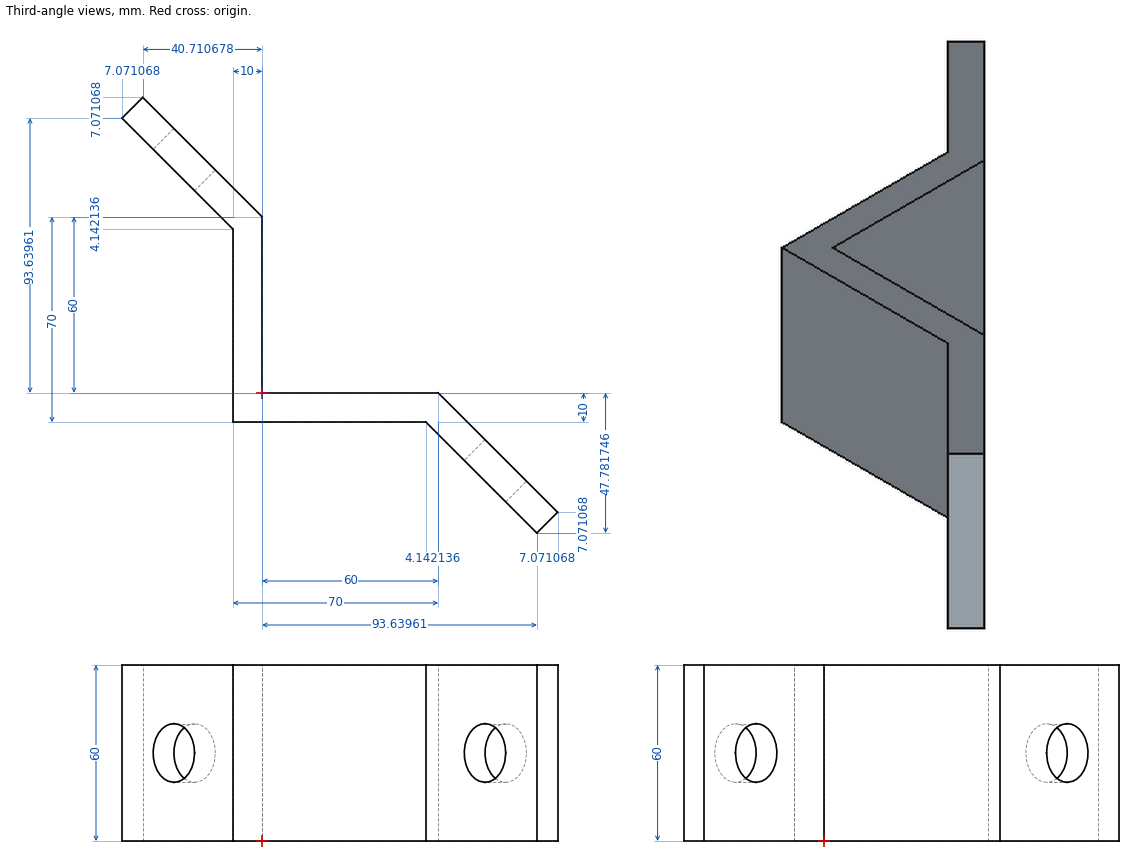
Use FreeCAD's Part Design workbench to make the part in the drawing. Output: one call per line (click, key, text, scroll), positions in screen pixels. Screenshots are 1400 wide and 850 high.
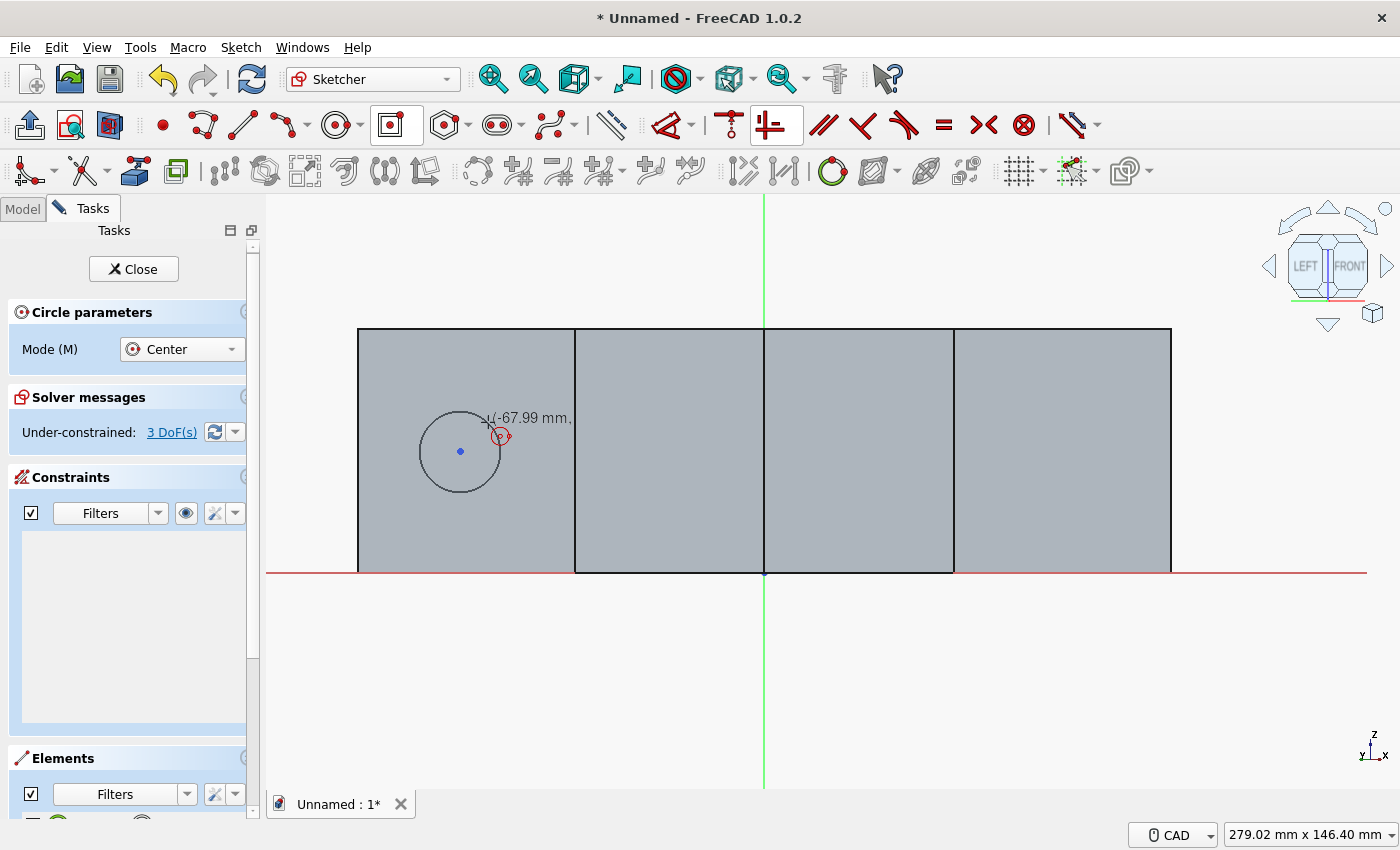
click(1069, 451)
click(1098, 422)
key(Escape)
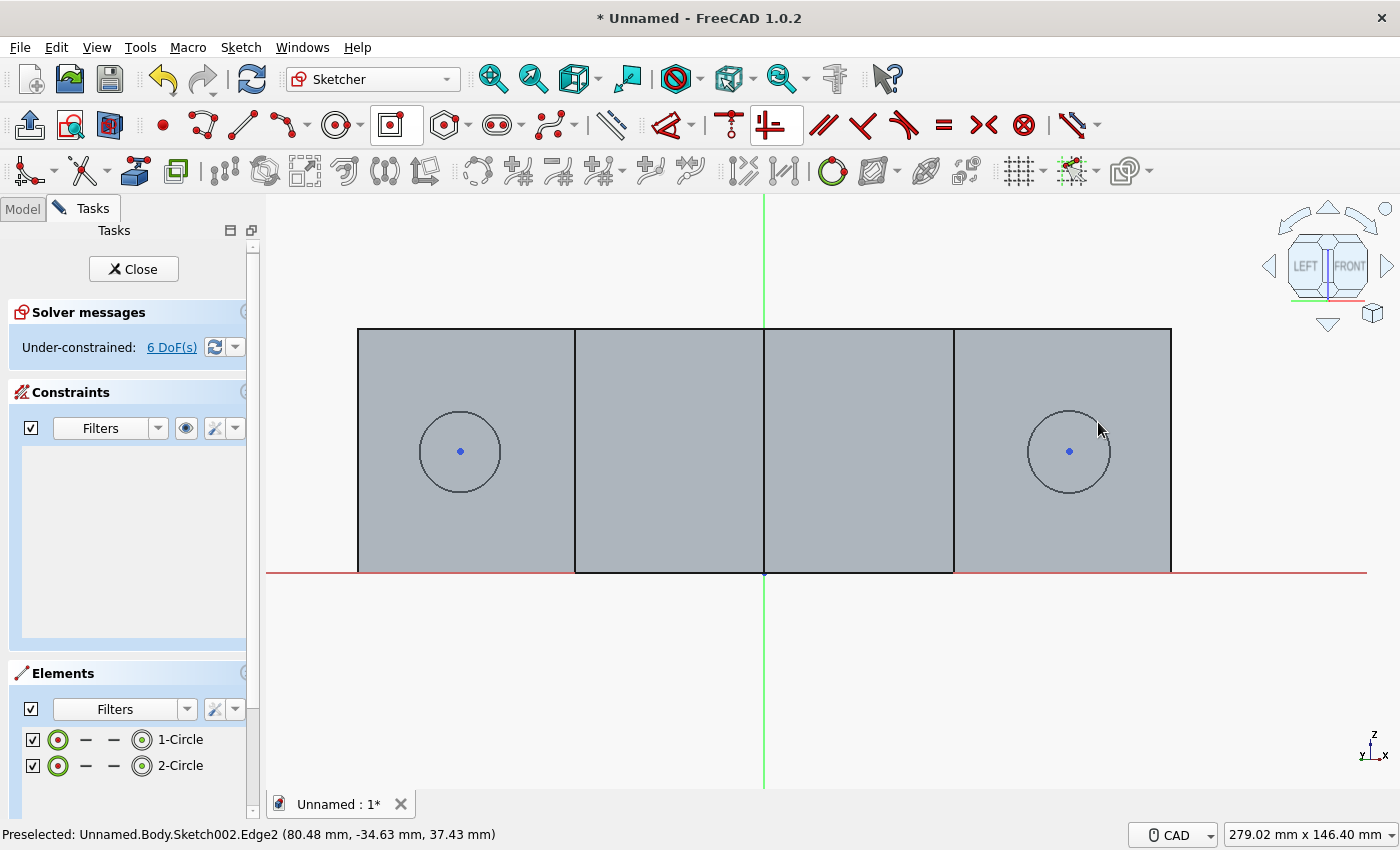
click(488, 423)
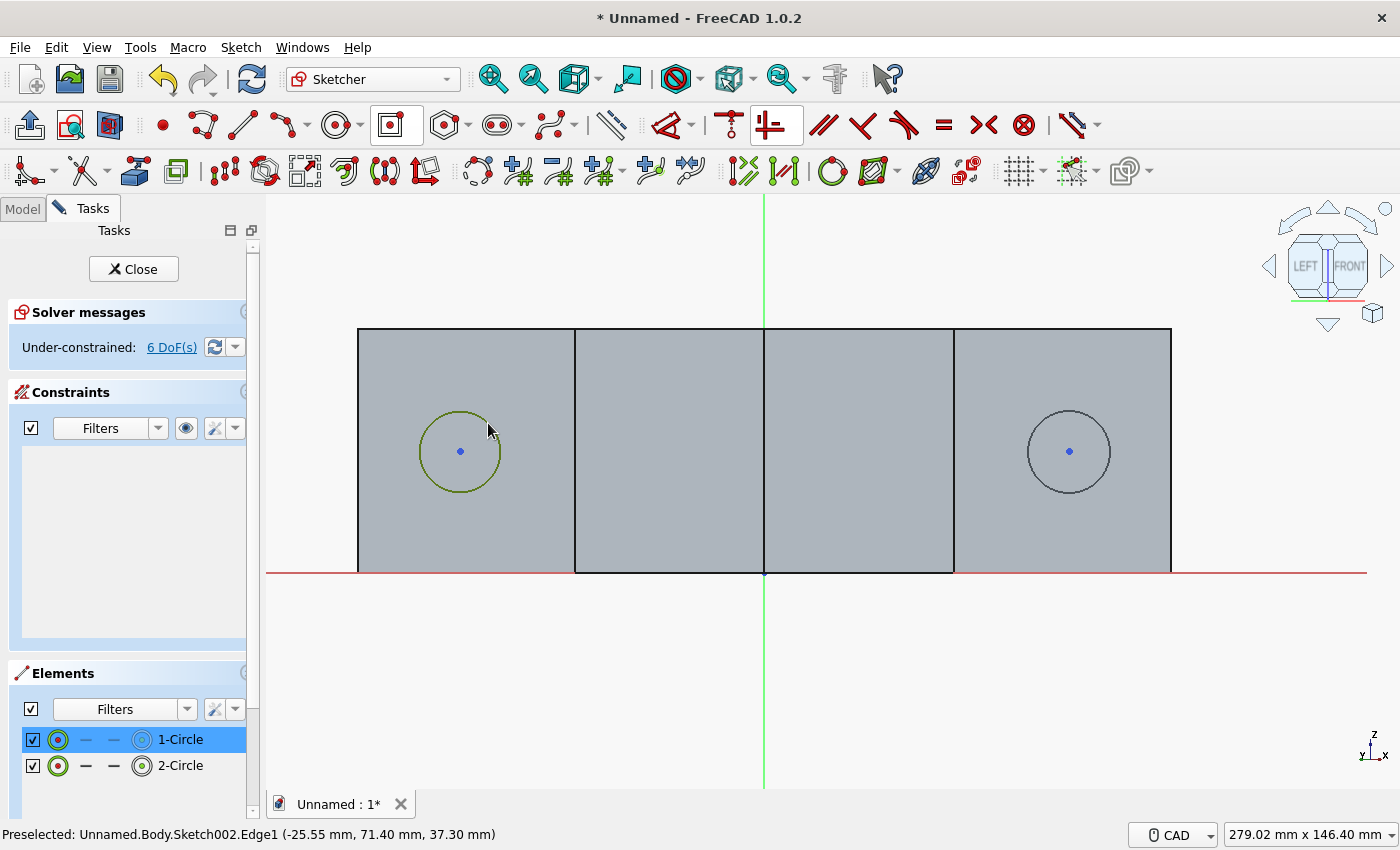
click(1098, 423)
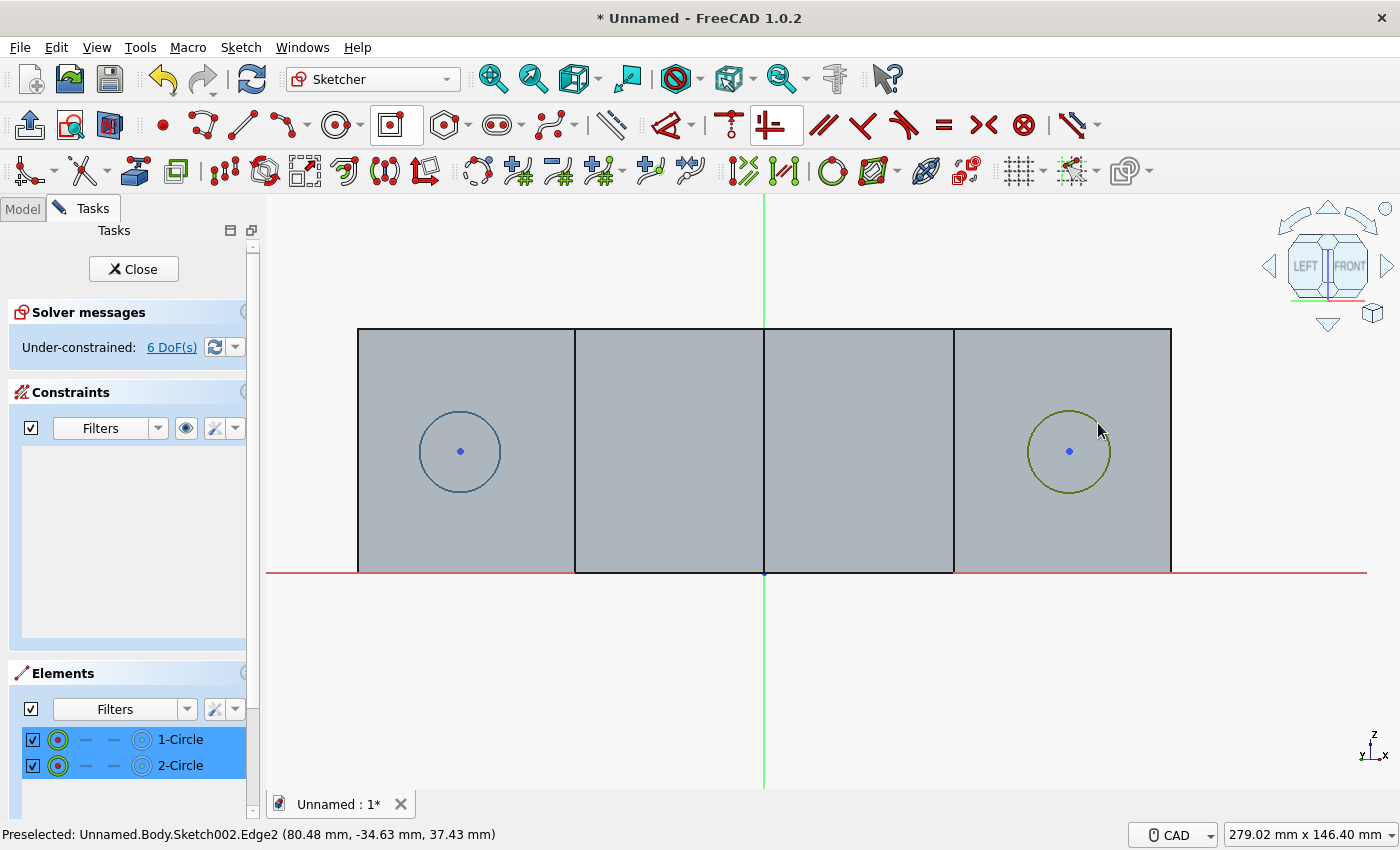
click(944, 126)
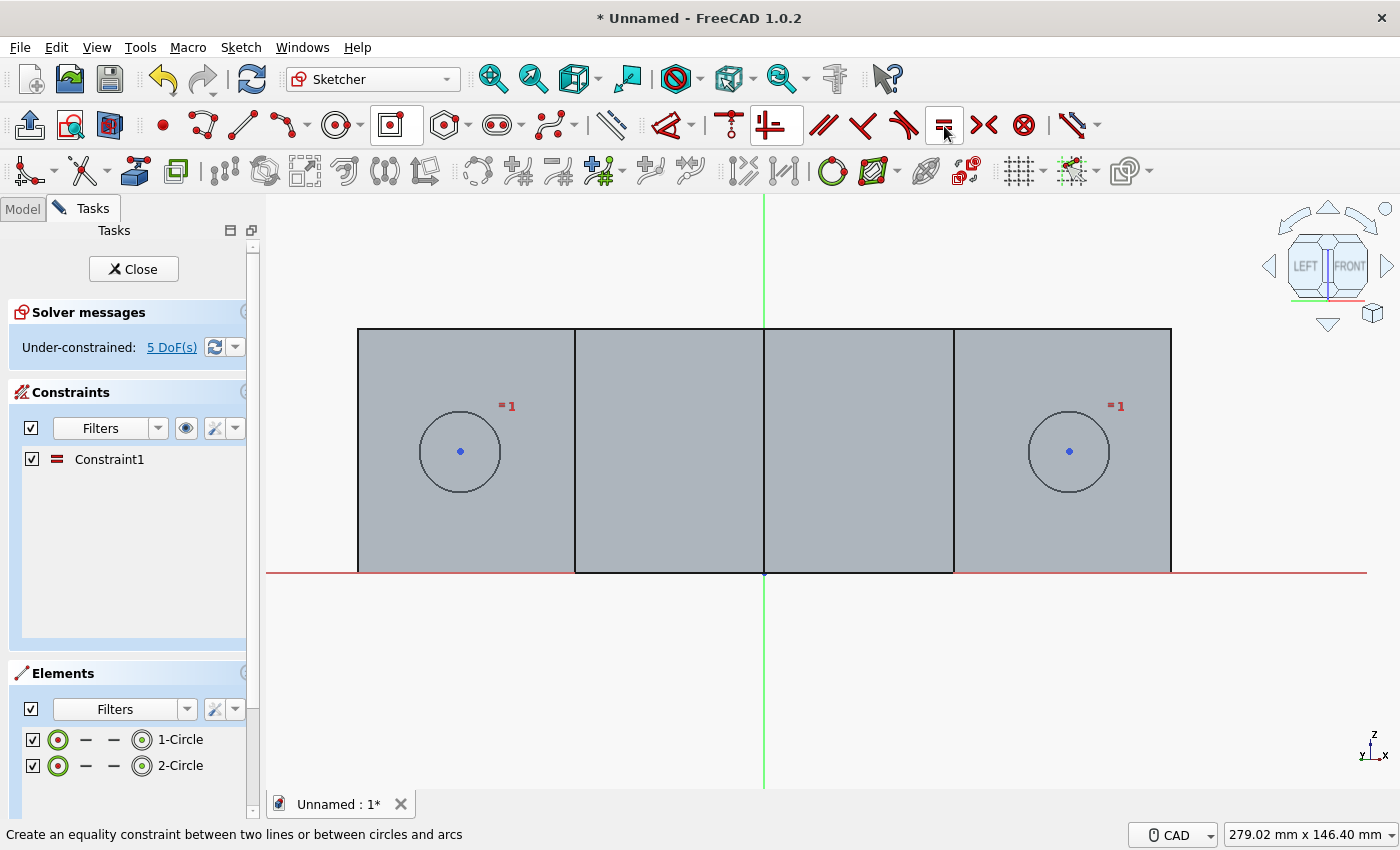
click(460, 452)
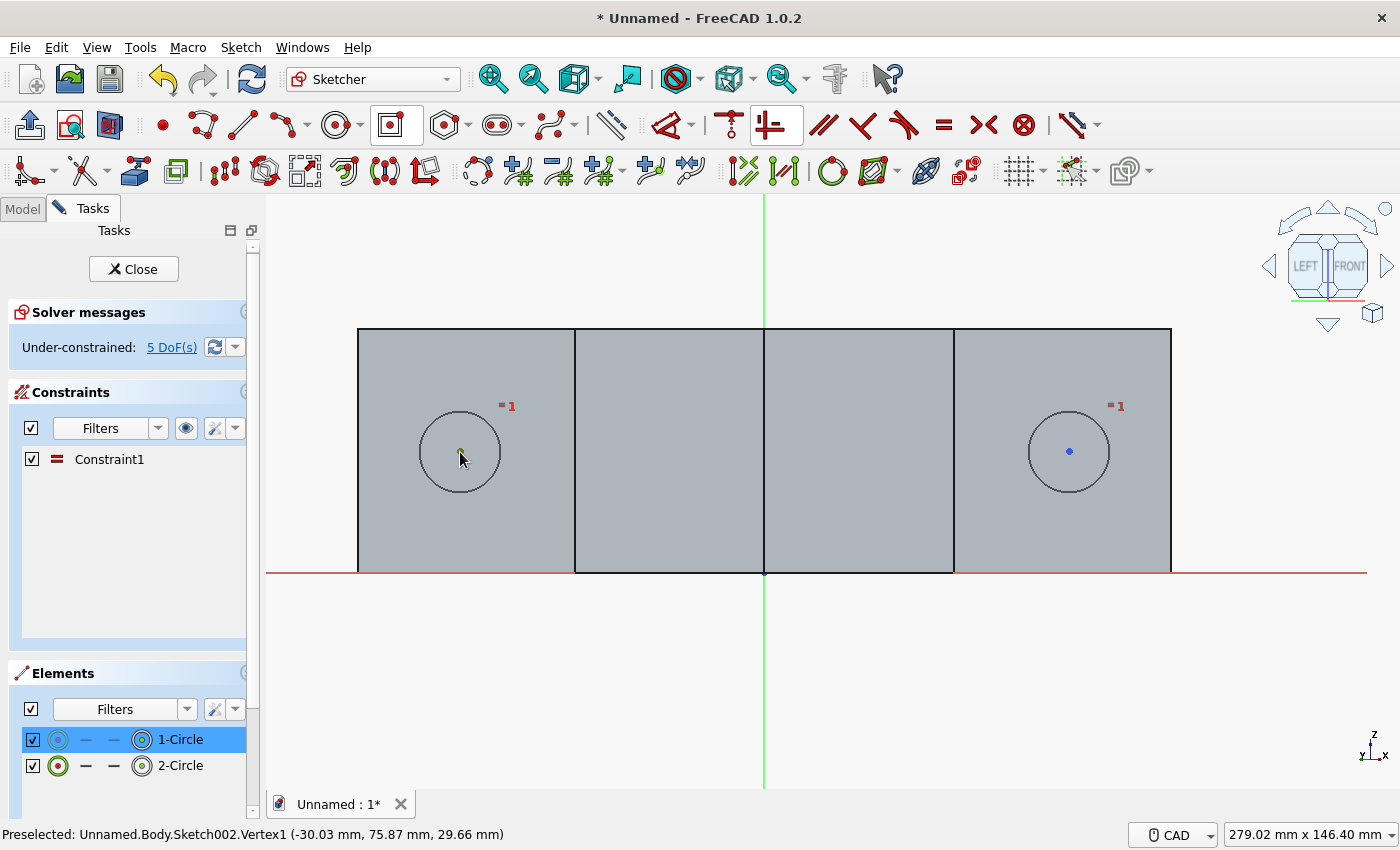
click(1069, 452)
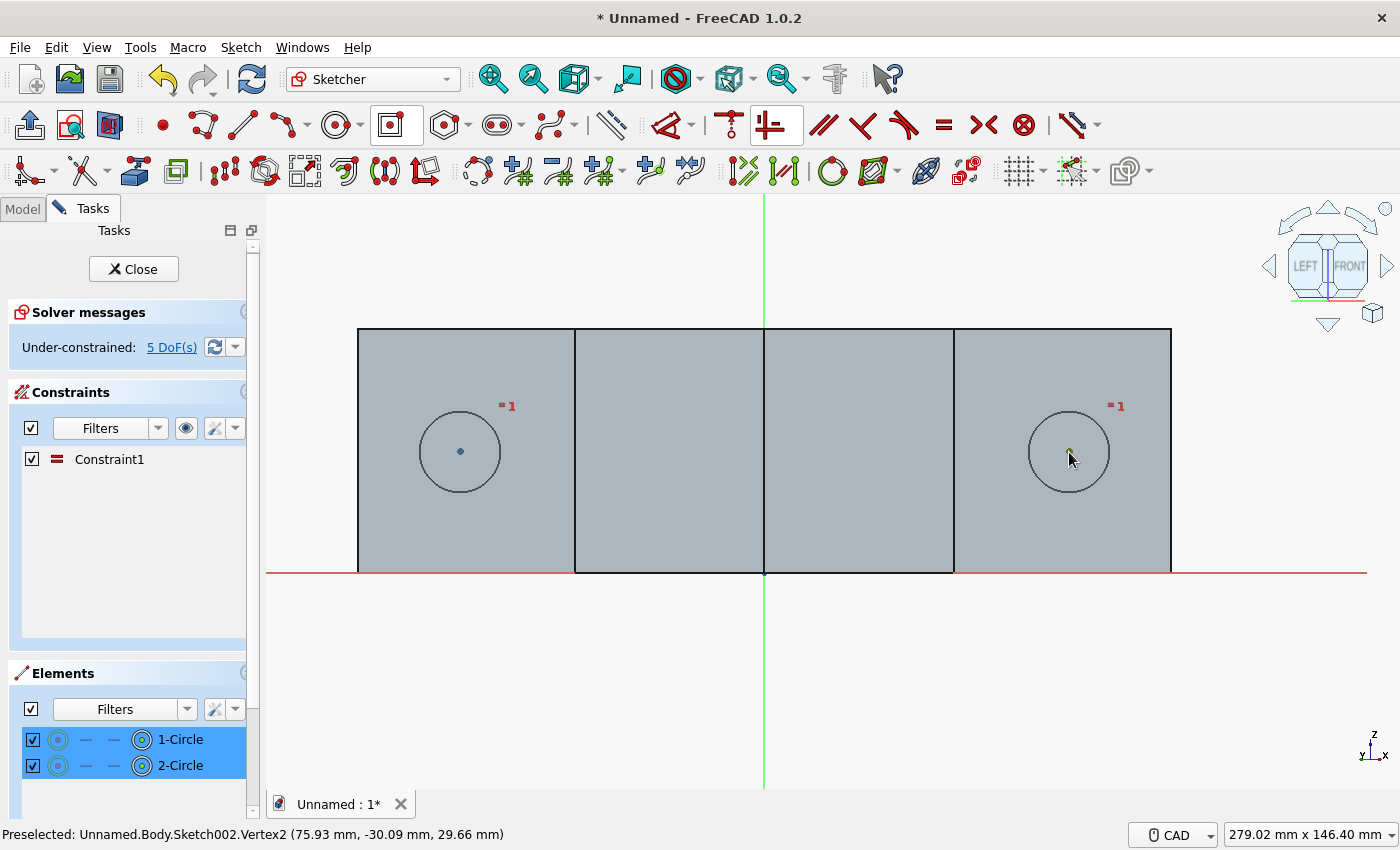
click(798, 126)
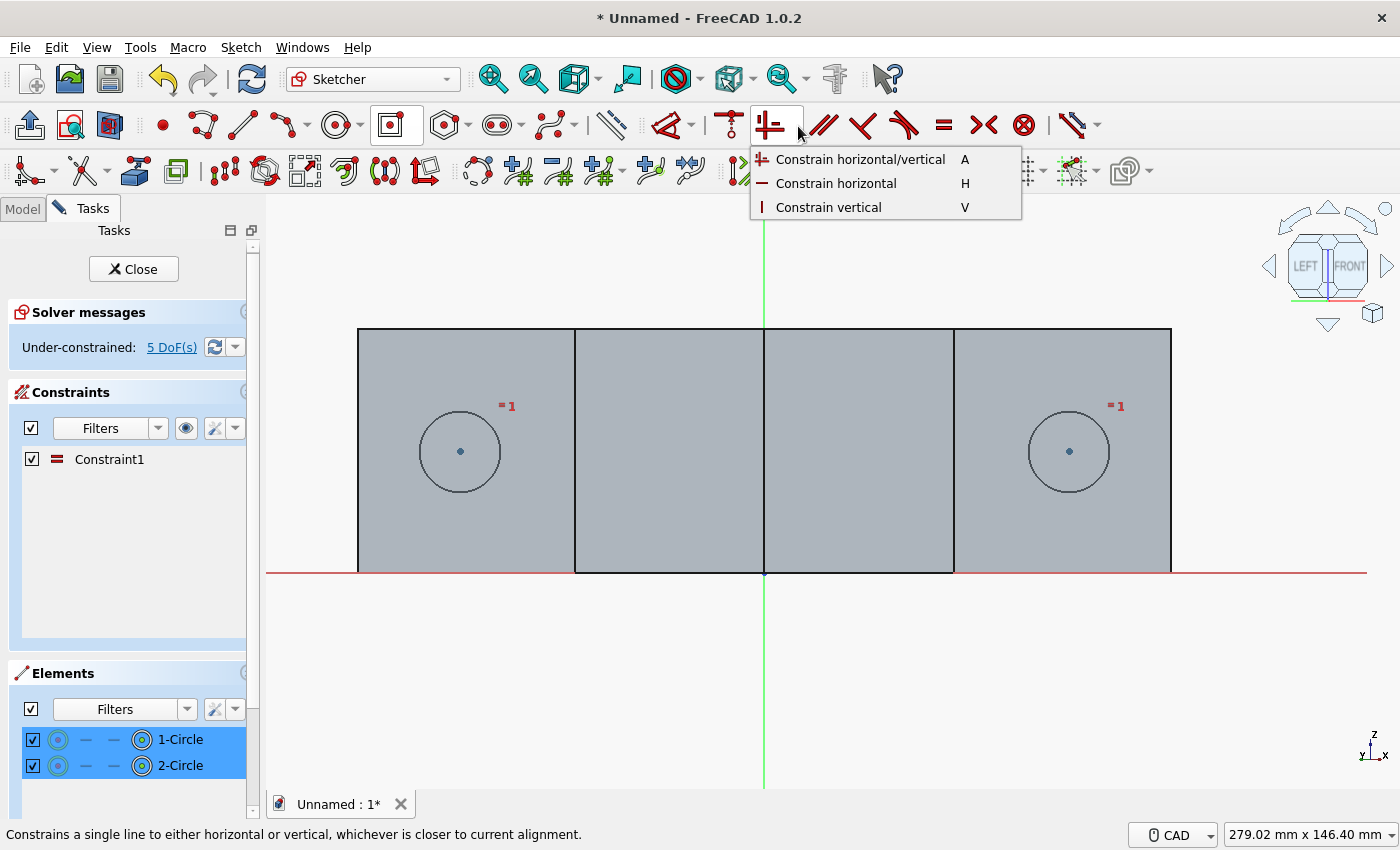
click(886, 183)